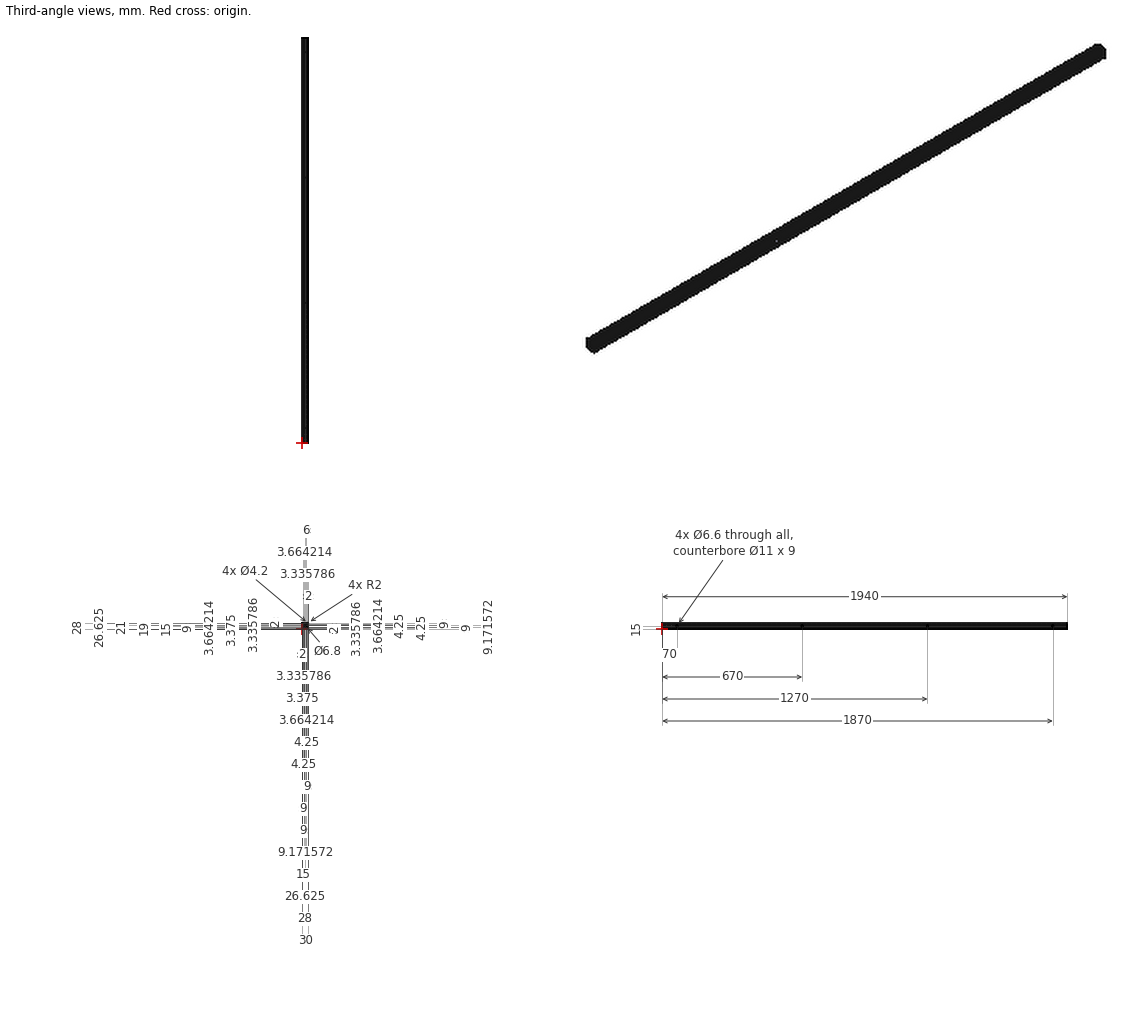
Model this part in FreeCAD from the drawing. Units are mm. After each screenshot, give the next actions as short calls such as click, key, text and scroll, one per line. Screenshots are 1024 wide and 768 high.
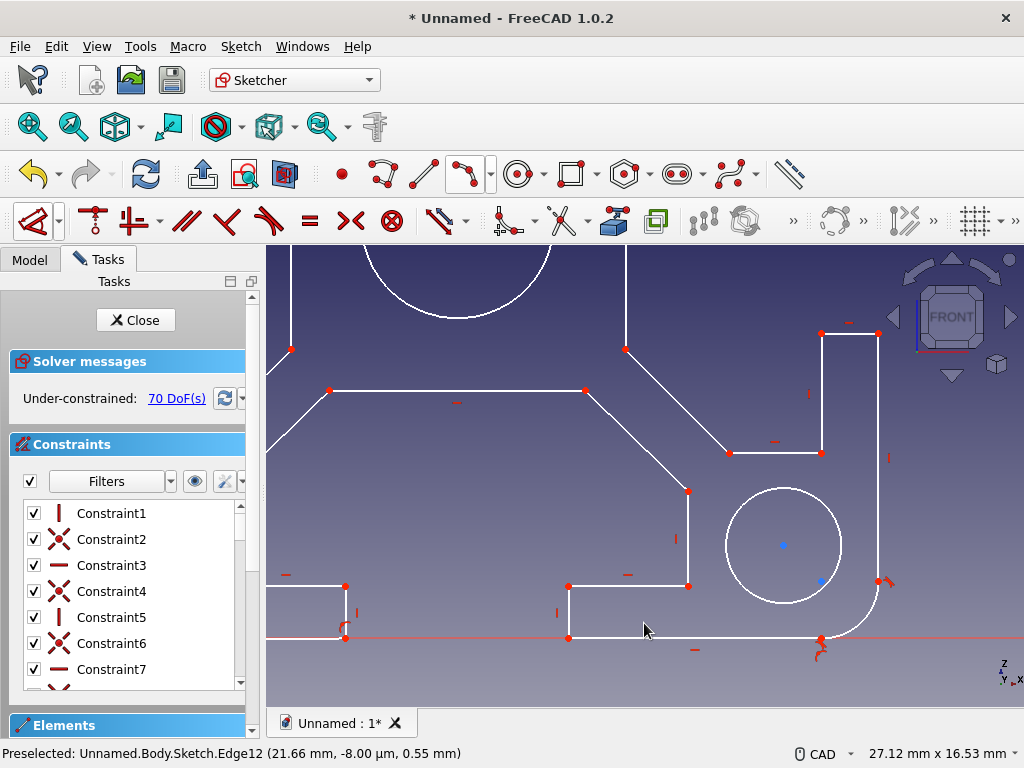
click(295, 639)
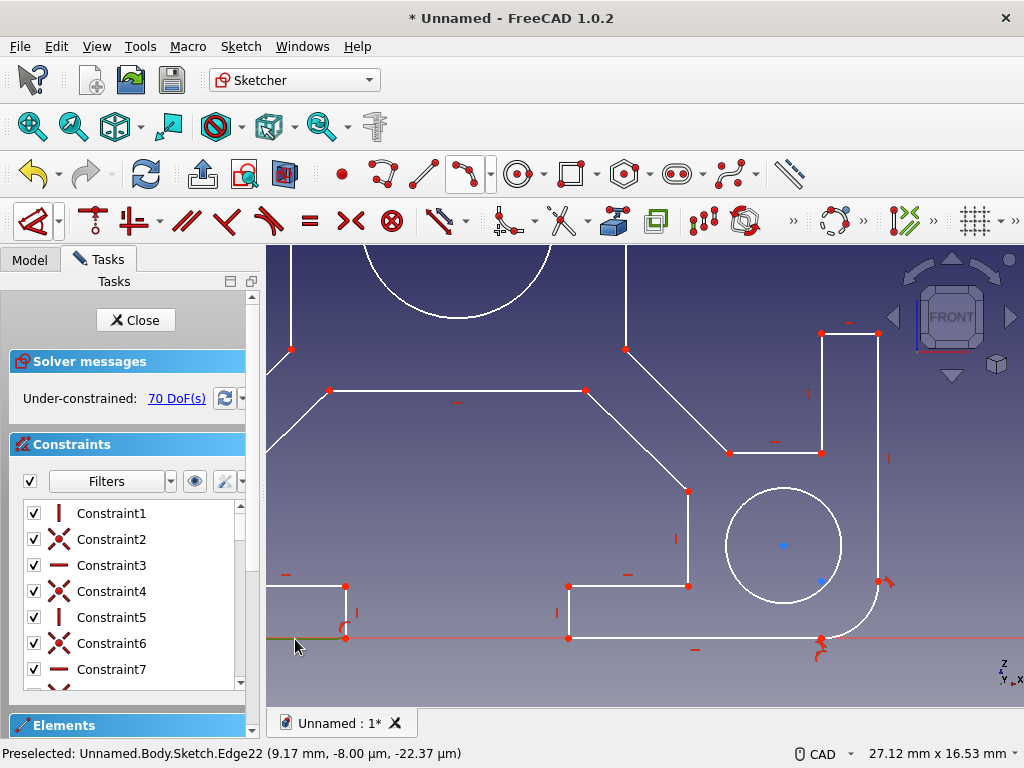
key(h)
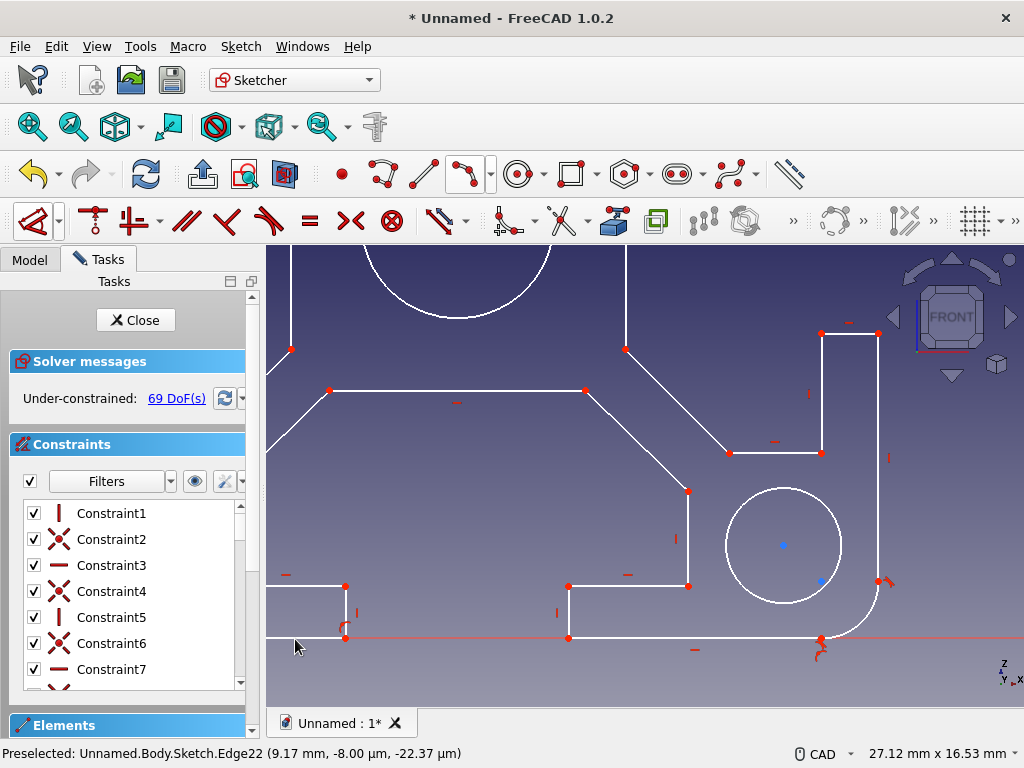
scroll(645, 625, down, 5)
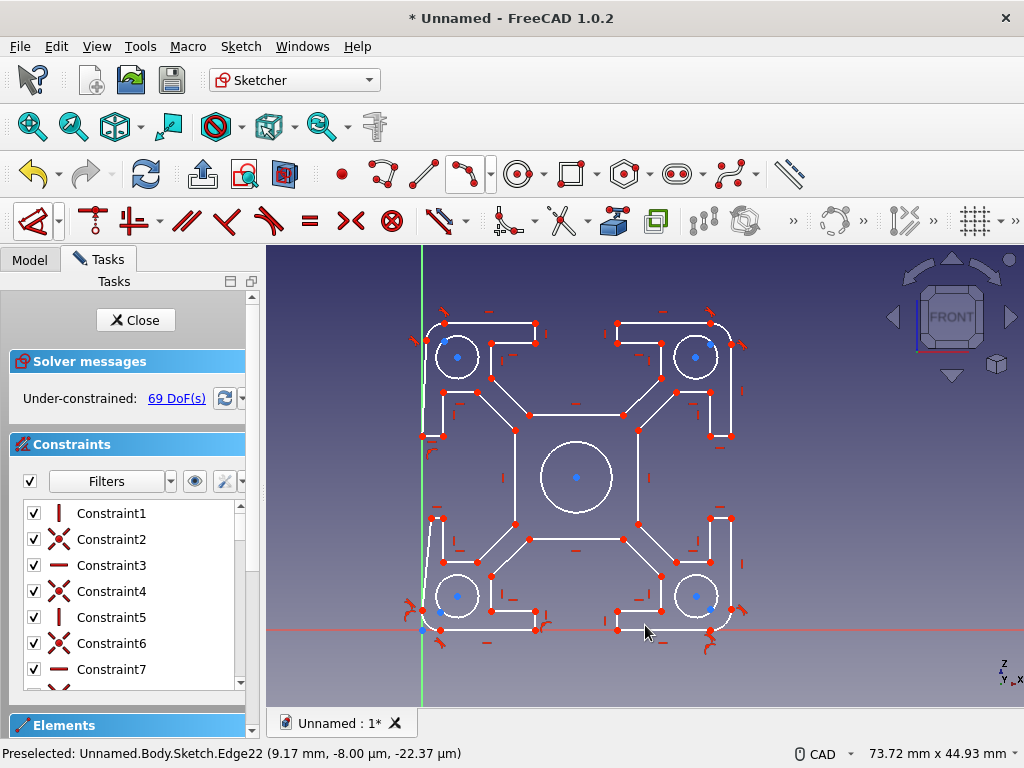
scroll(429, 546, up, 4)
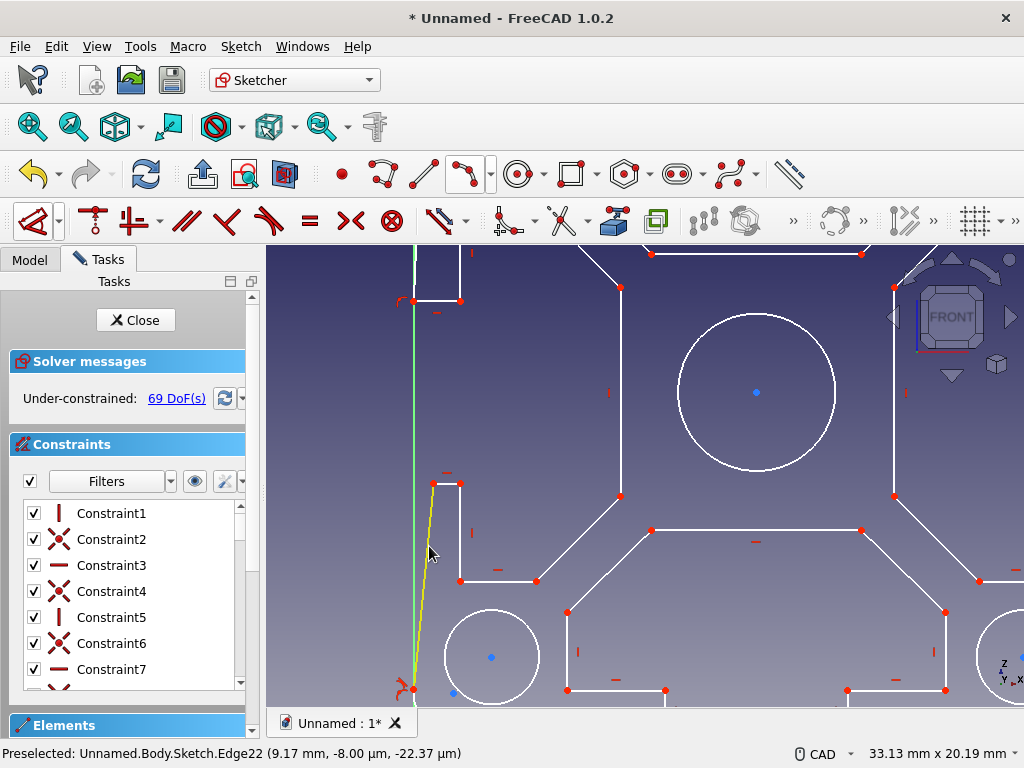
click(428, 545)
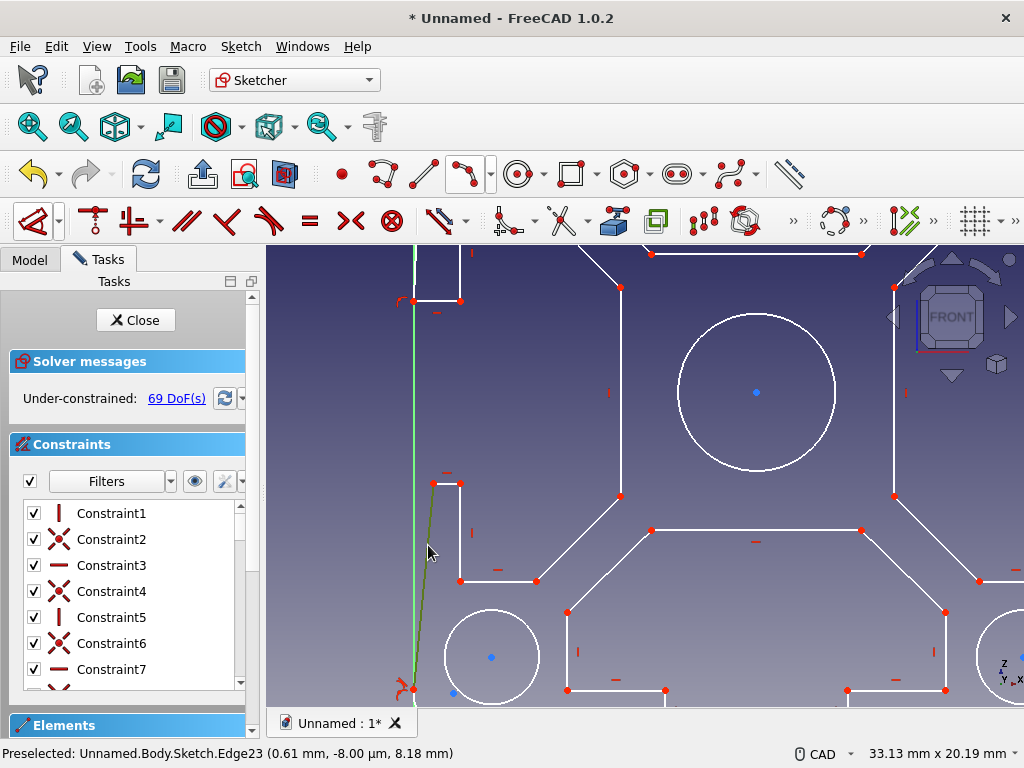
key(v)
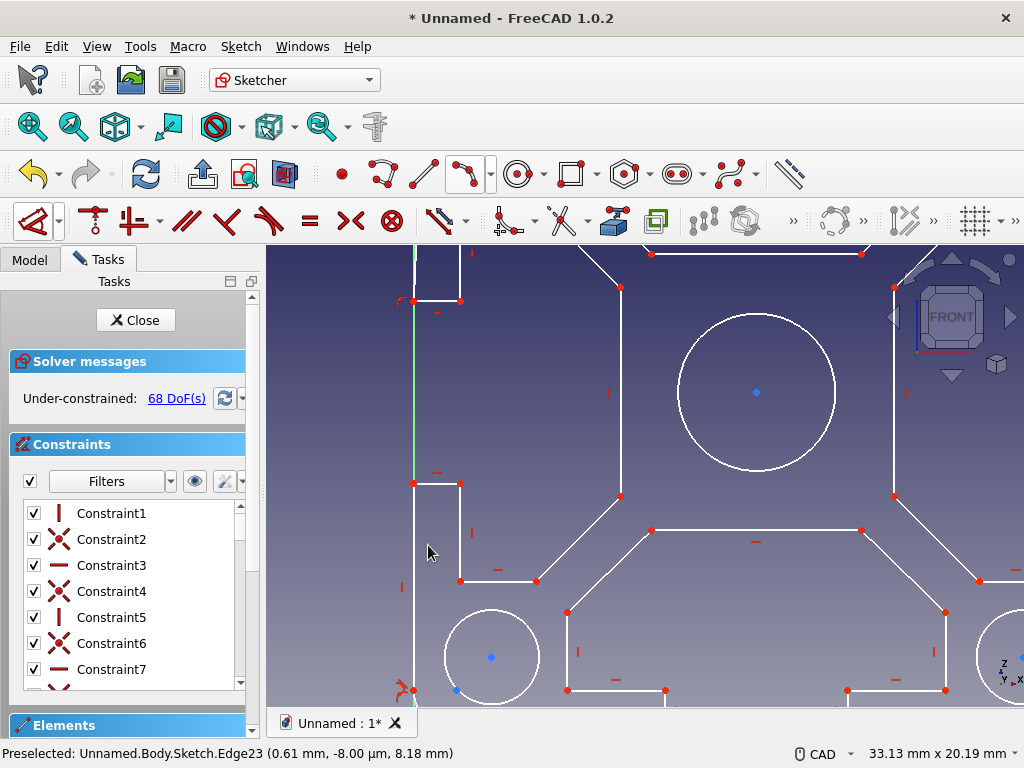
scroll(429, 546, down, 4)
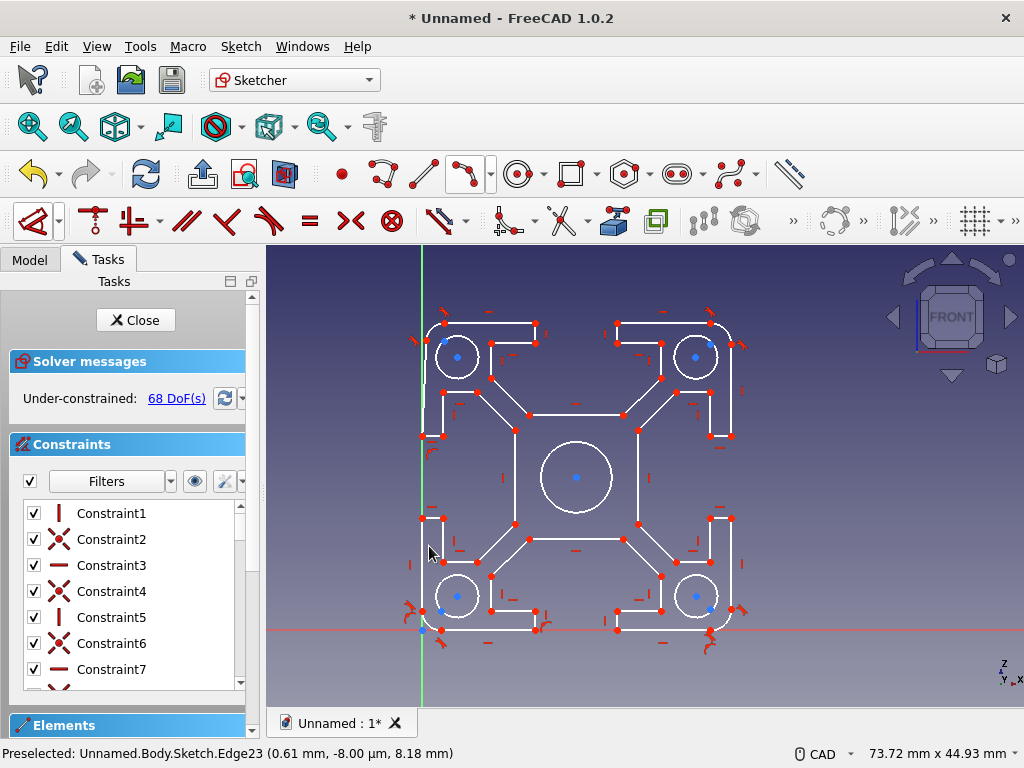
click(423, 408)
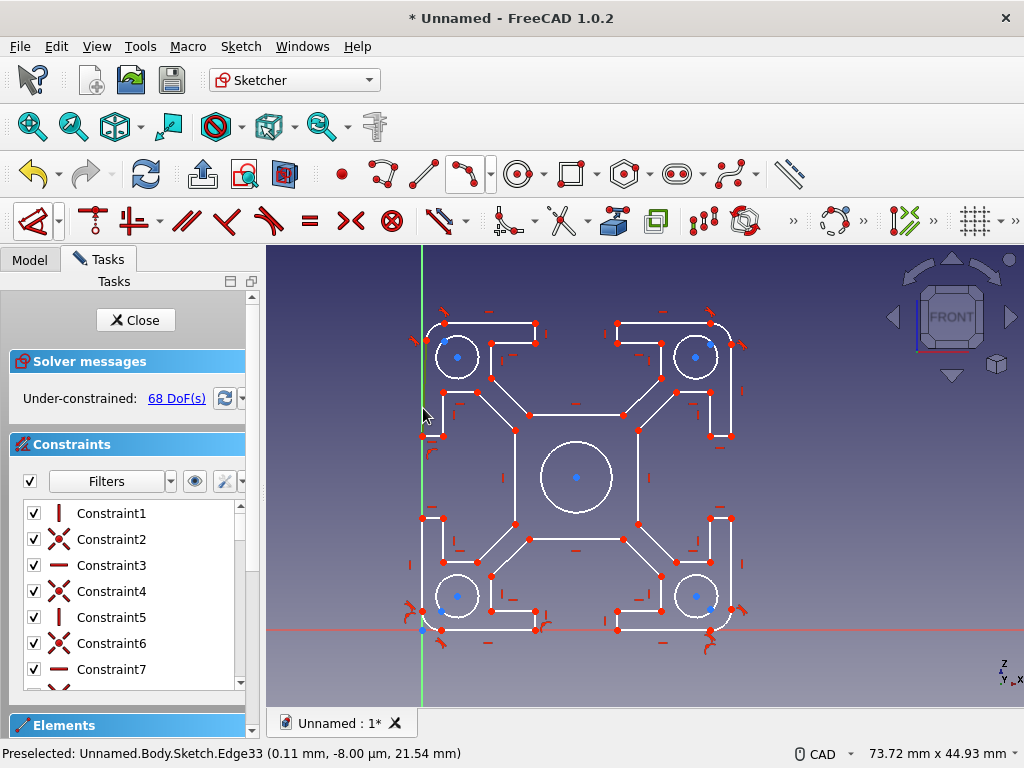
key(v)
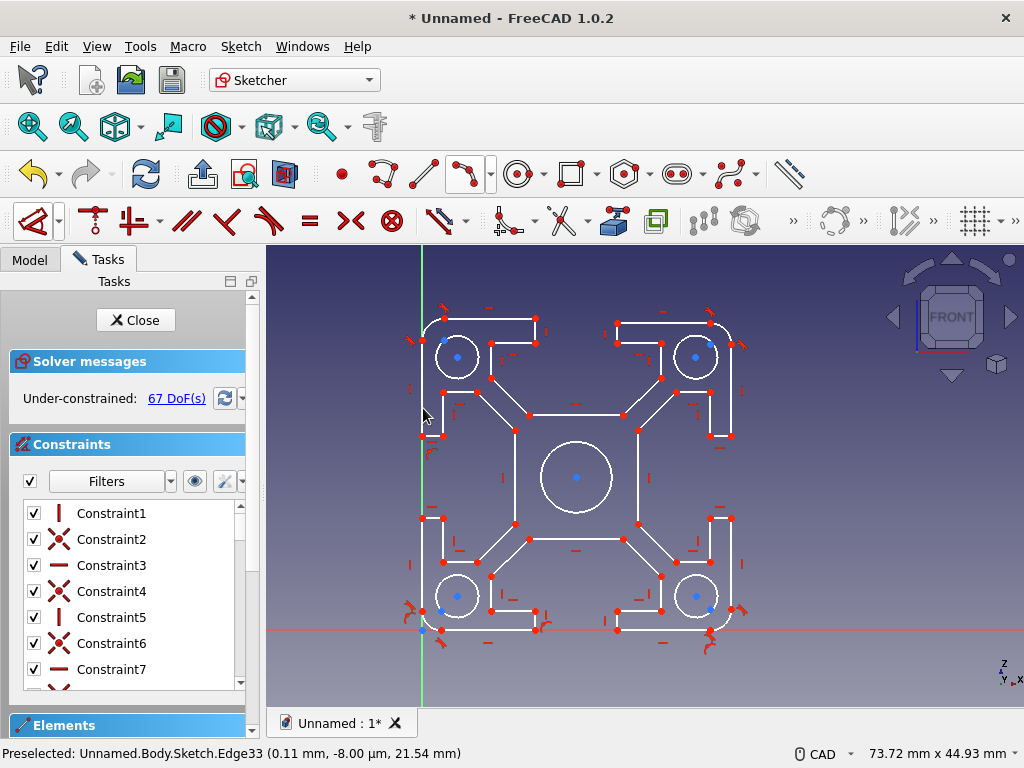
scroll(720, 628, up, 2)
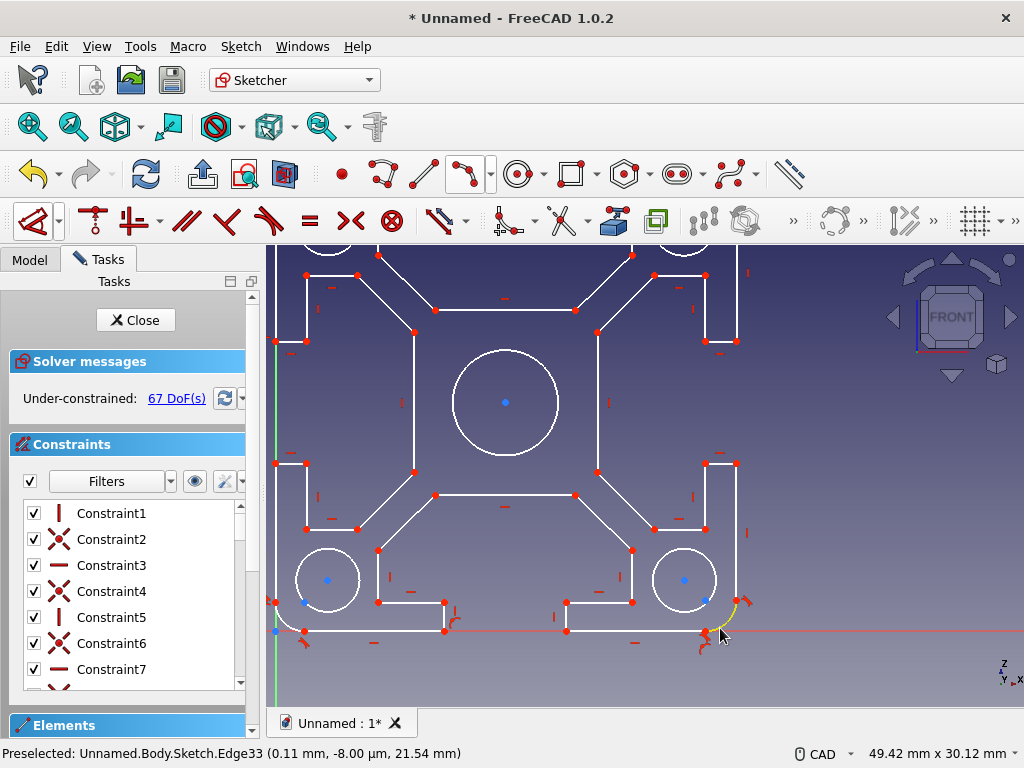
click(719, 628)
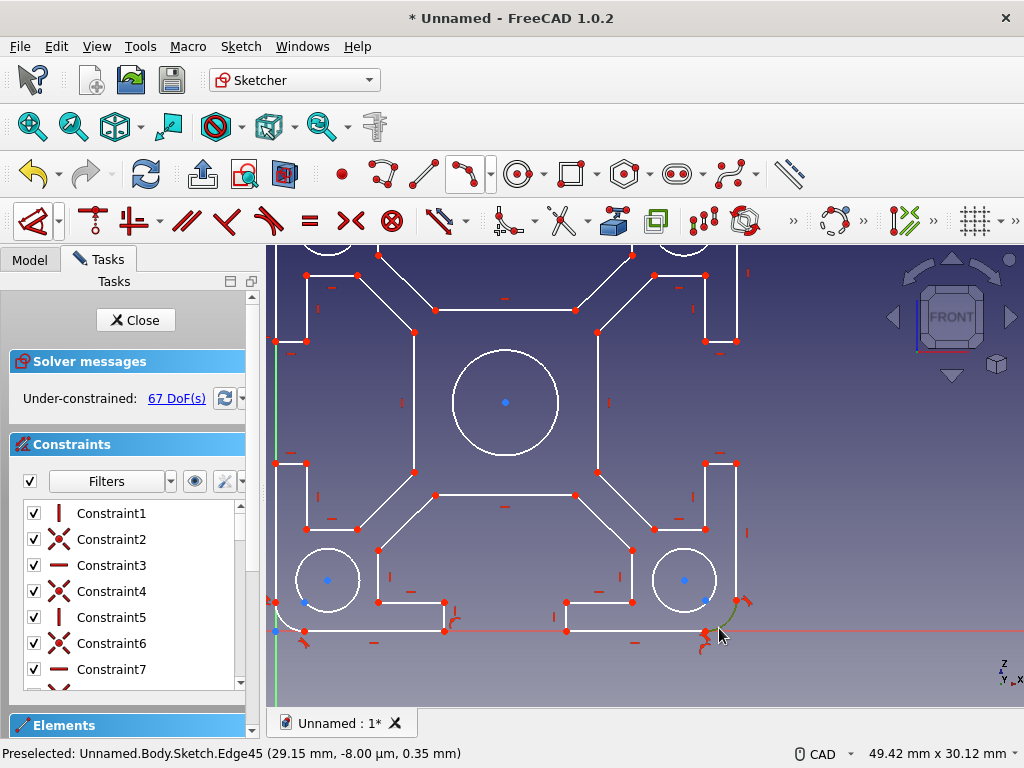
scroll(296, 630, up, 3)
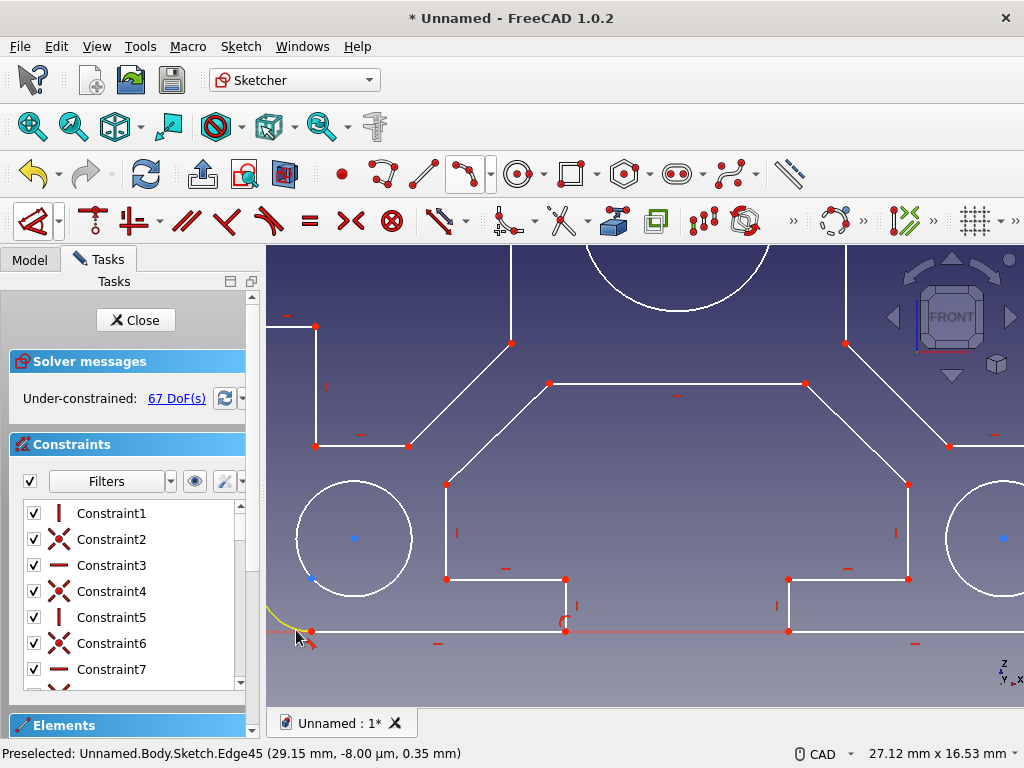
click(295, 629)